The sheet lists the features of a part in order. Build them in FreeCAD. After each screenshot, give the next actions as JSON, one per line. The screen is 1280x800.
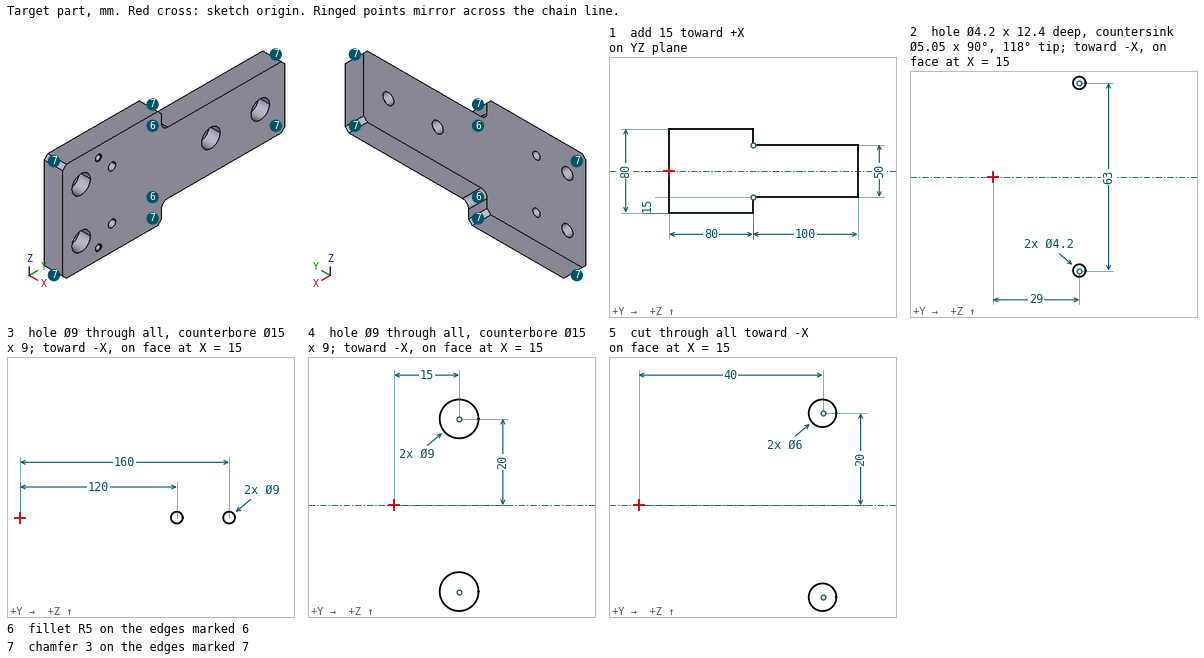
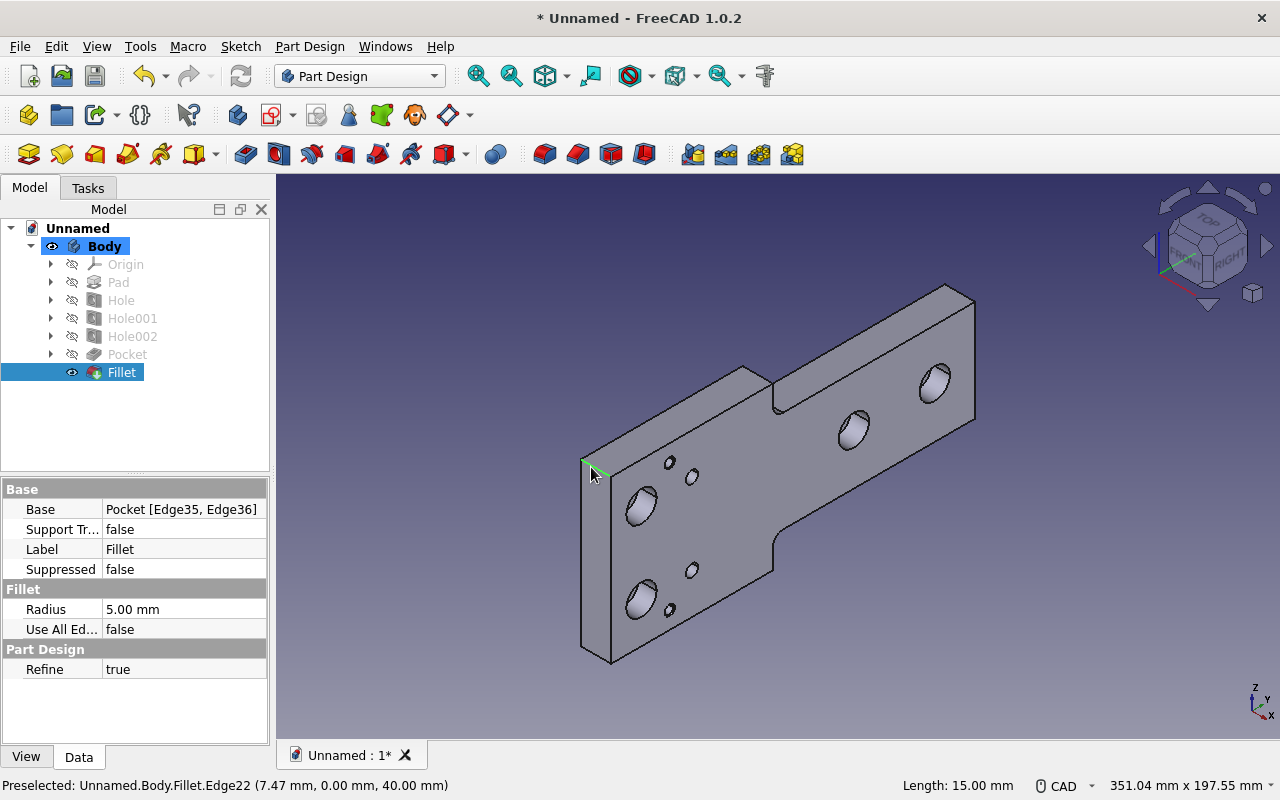
{"action": "key", "text": "2"}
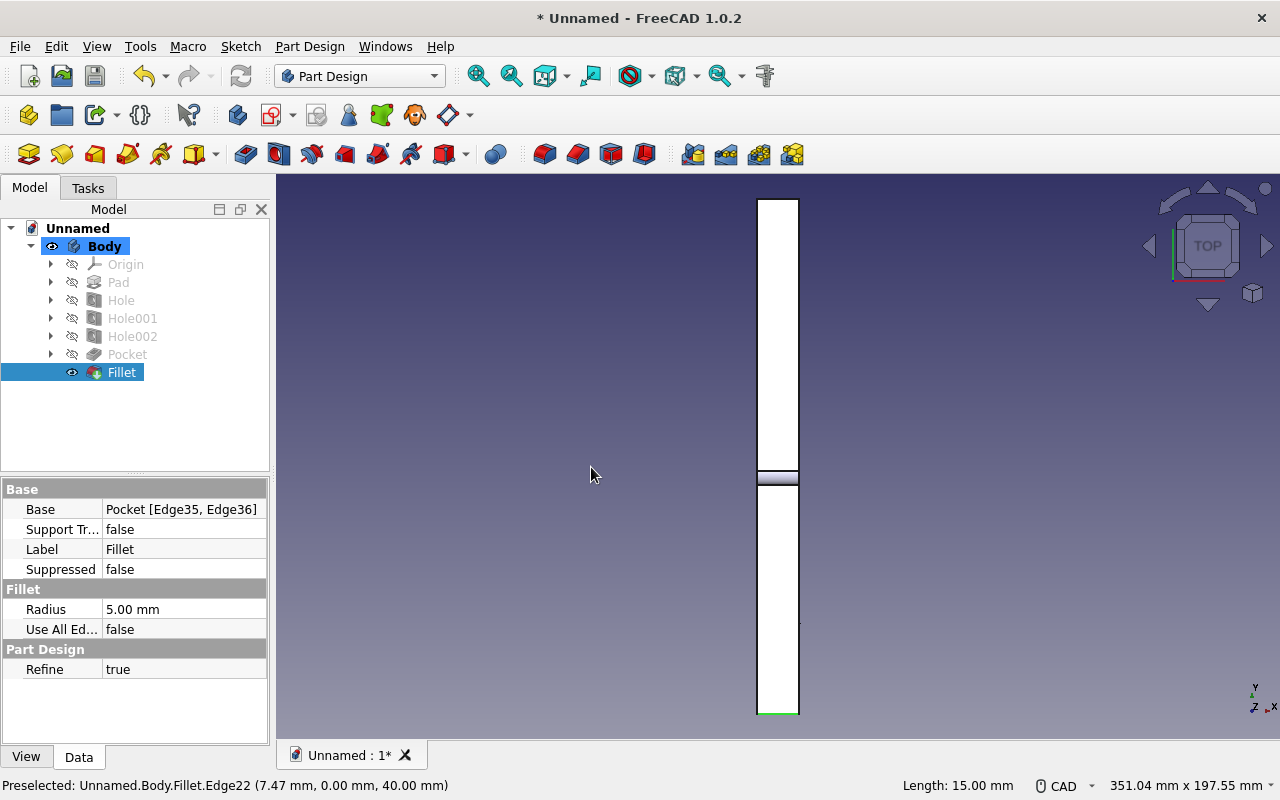
{"action": "left_click", "coordinate": [778, 484], "text": "ctrl"}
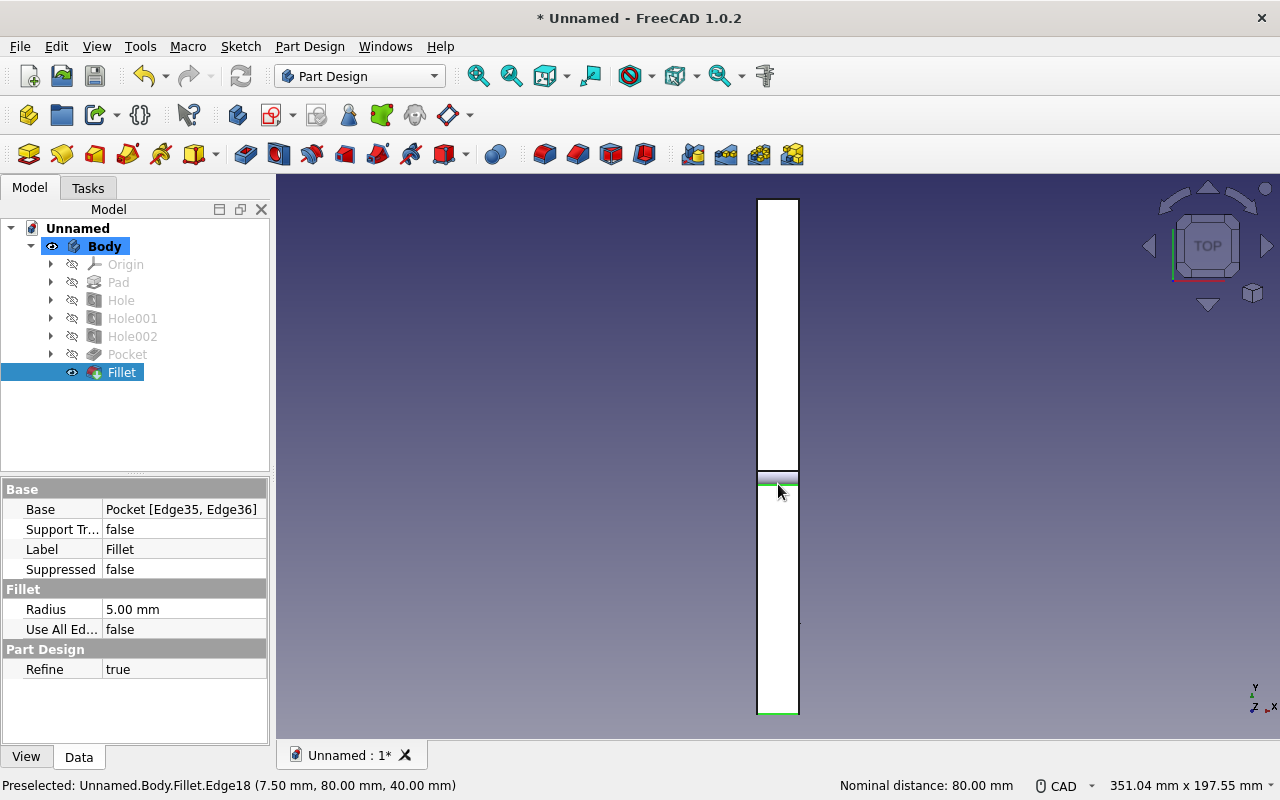
{"action": "key", "text": "0"}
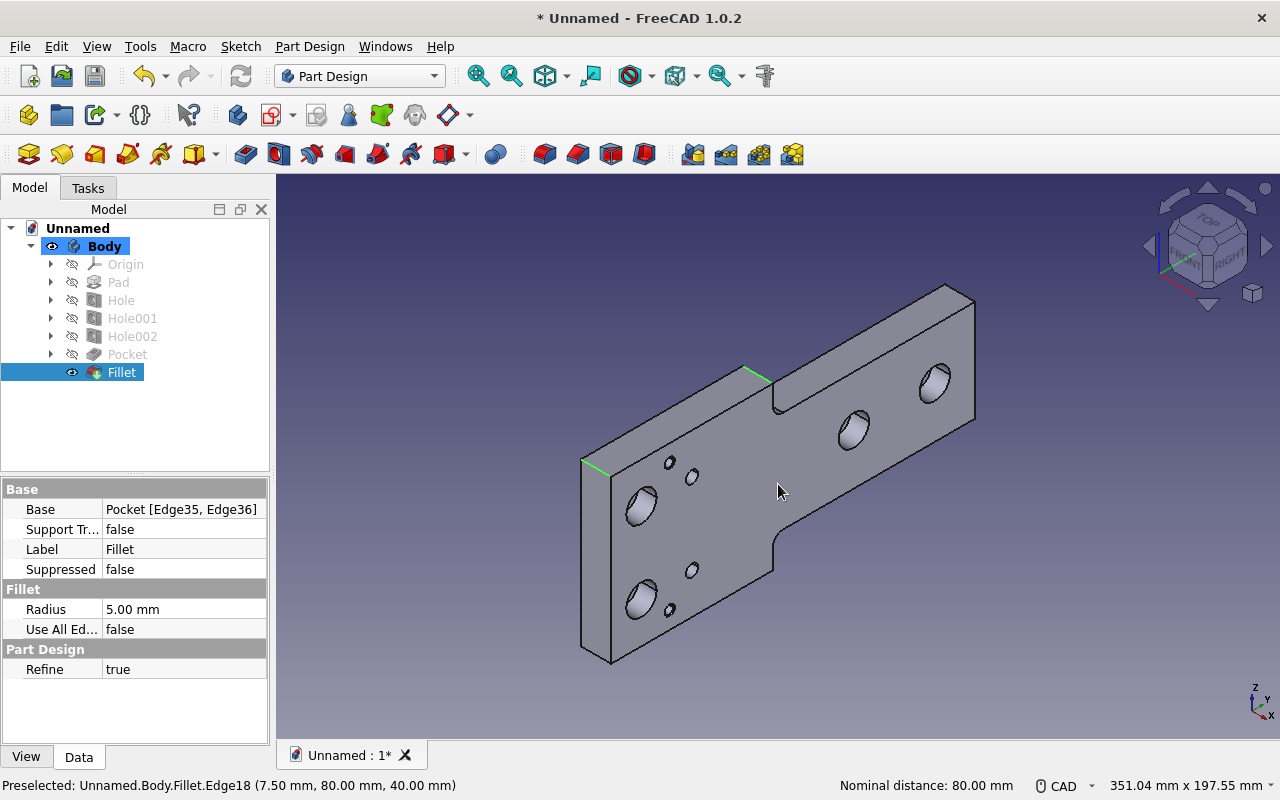
{"action": "key", "text": "1"}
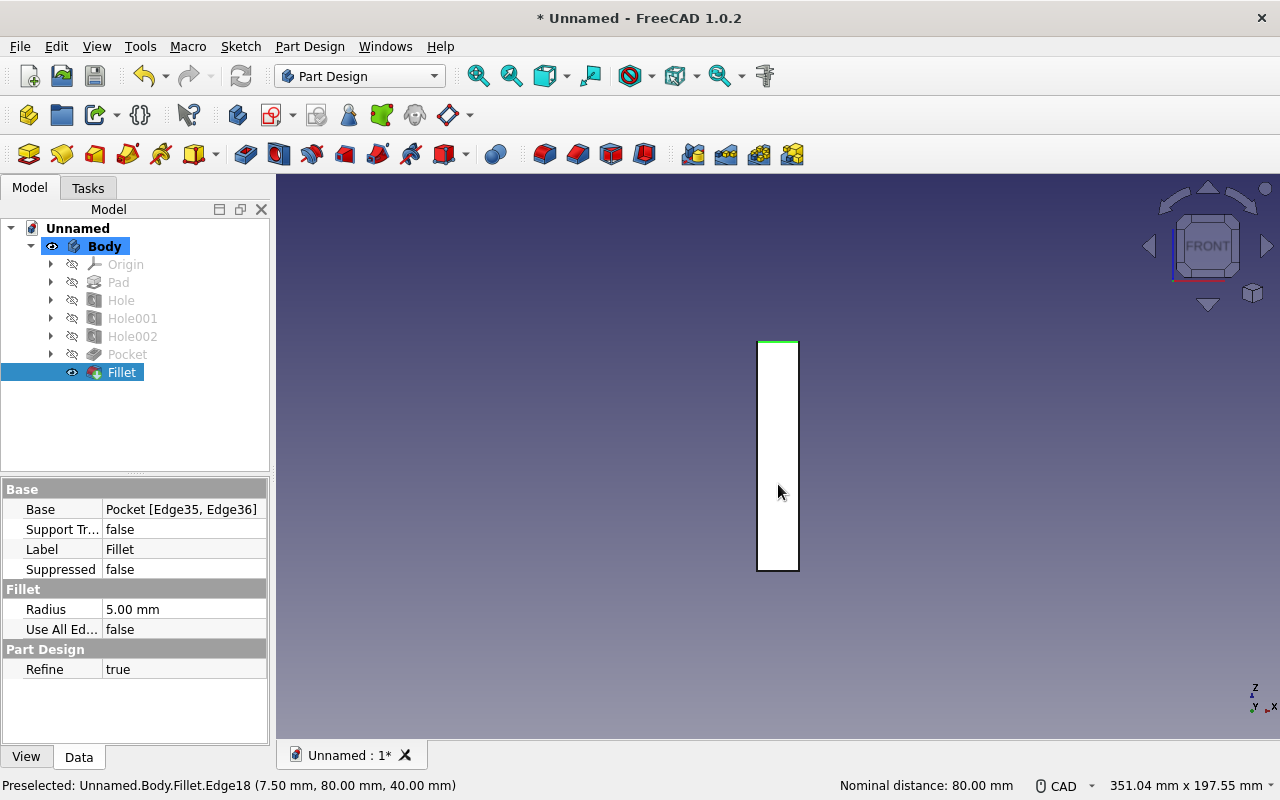
{"action": "left_click", "coordinate": [479, 76]}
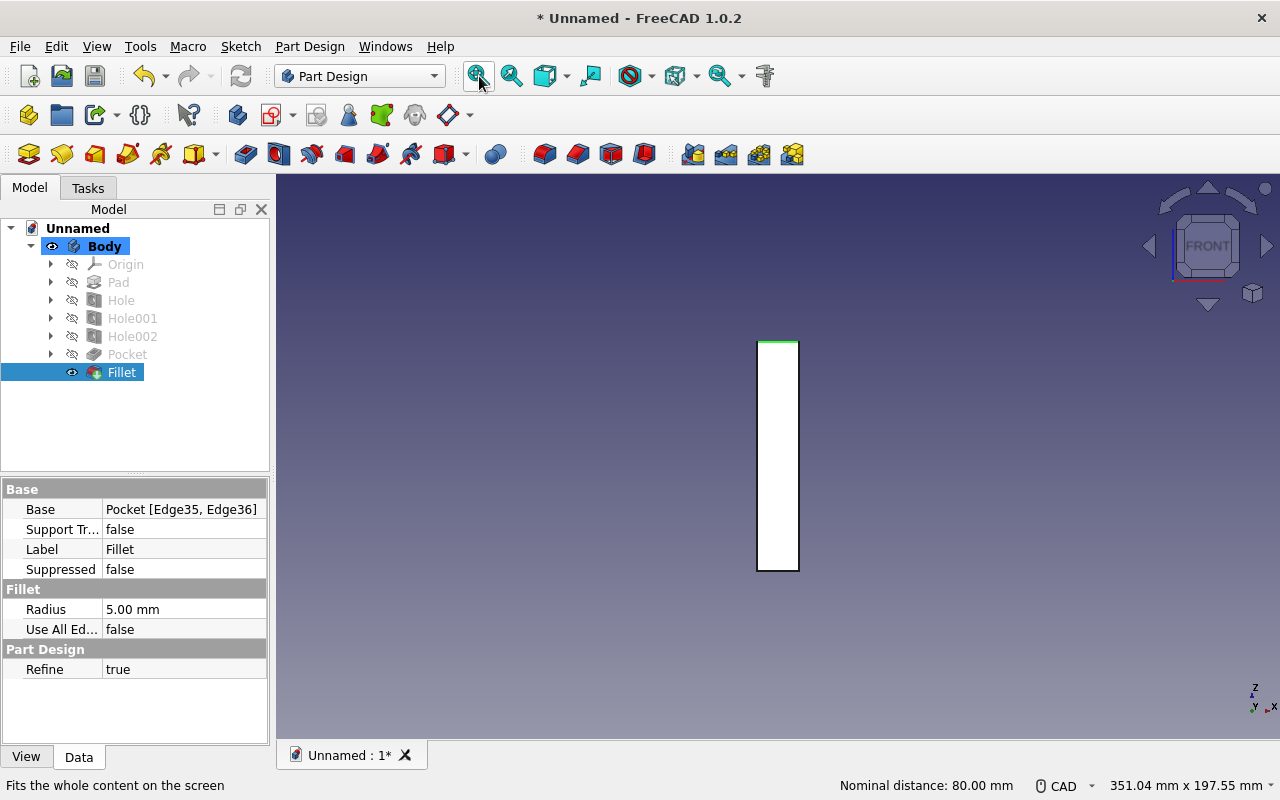
{"action": "left_click", "coordinate": [778, 570], "text": "ctrl"}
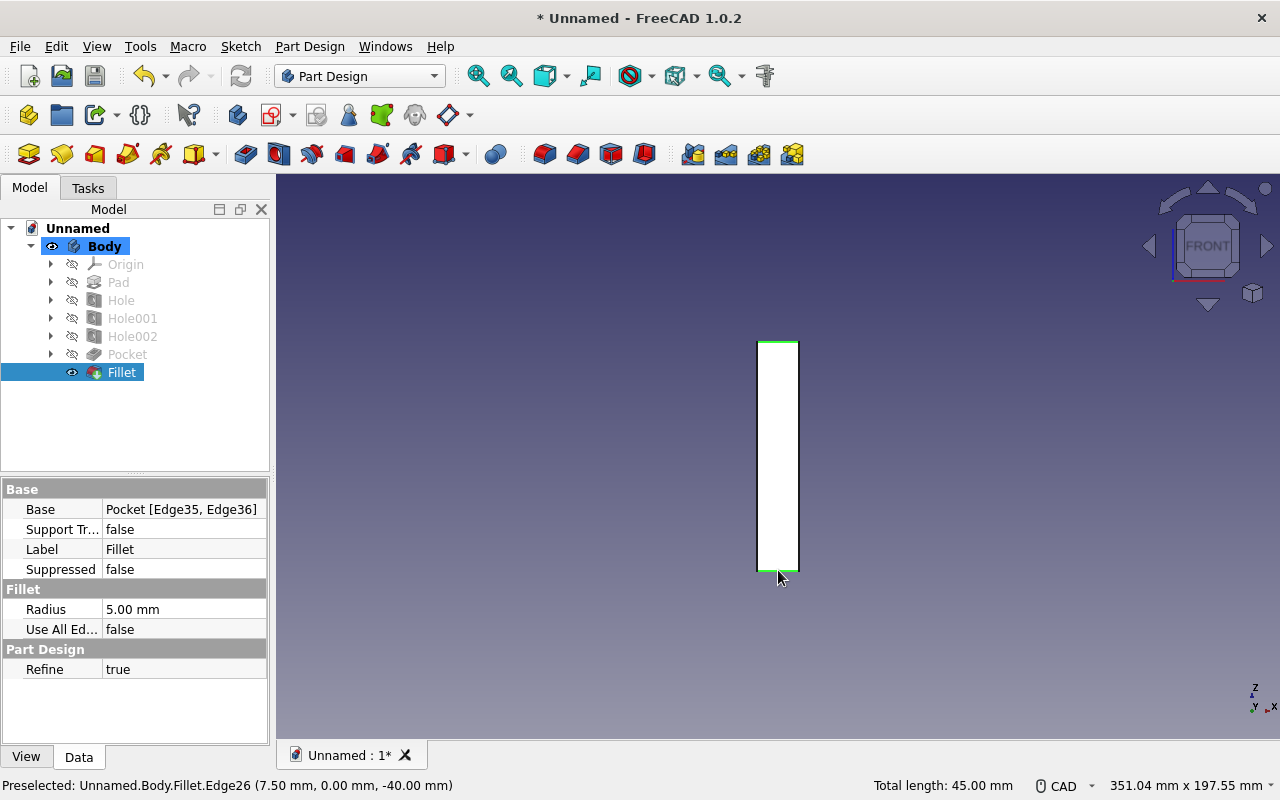
{"action": "key", "text": "3"}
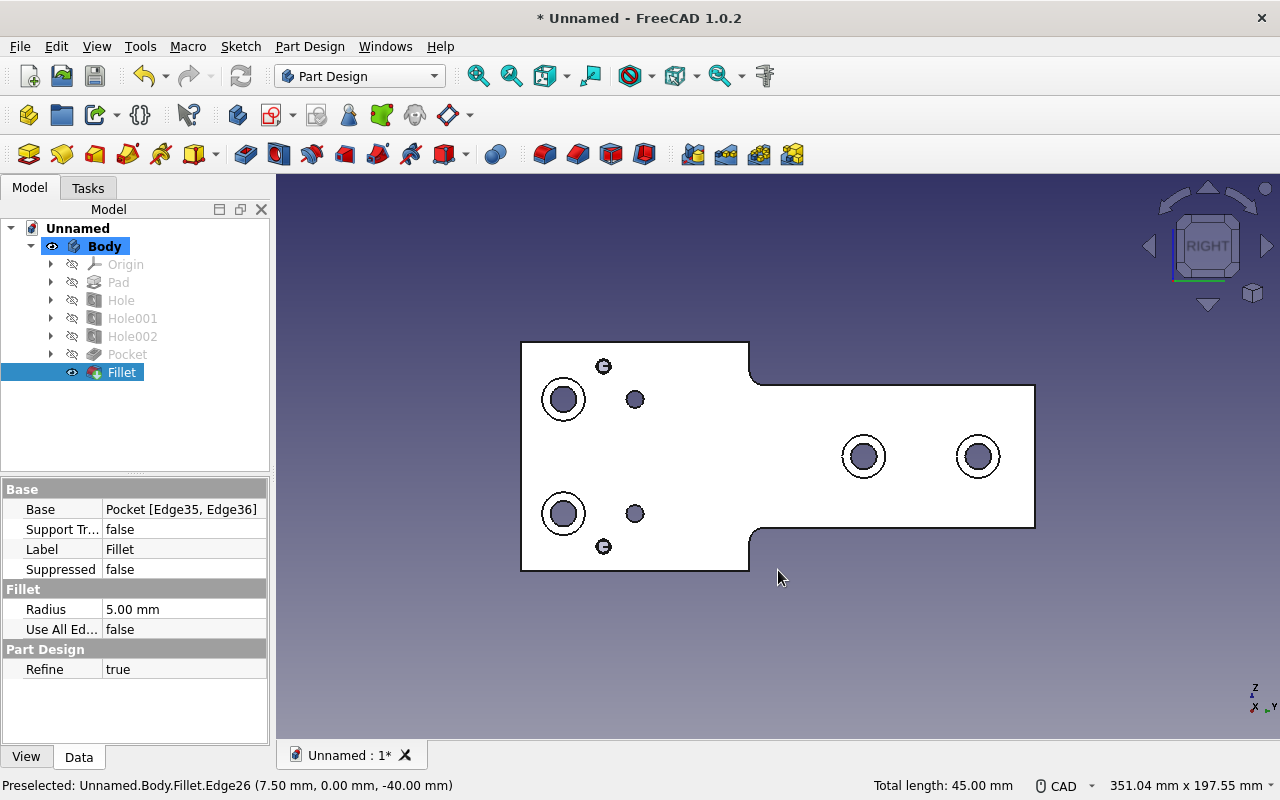
{"action": "key", "text": "5"}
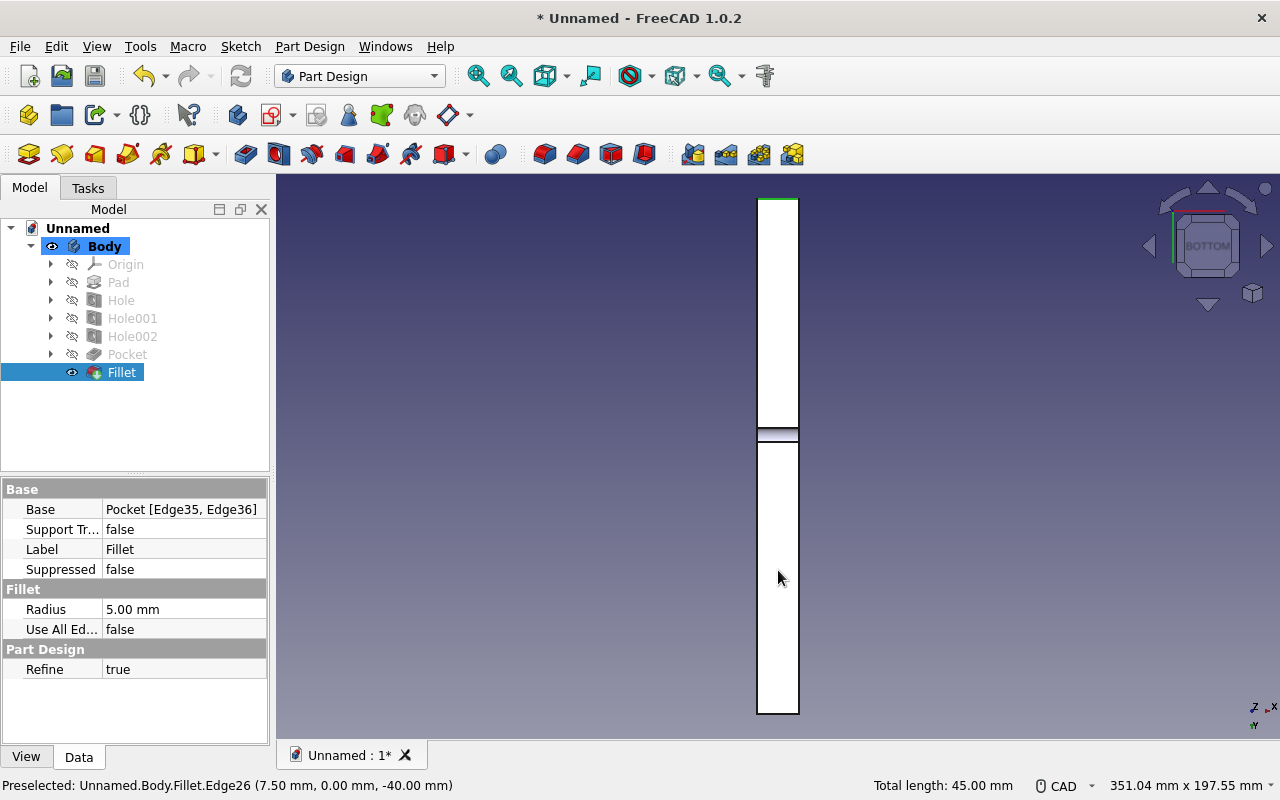
{"action": "left_click", "coordinate": [778, 427], "text": "ctrl"}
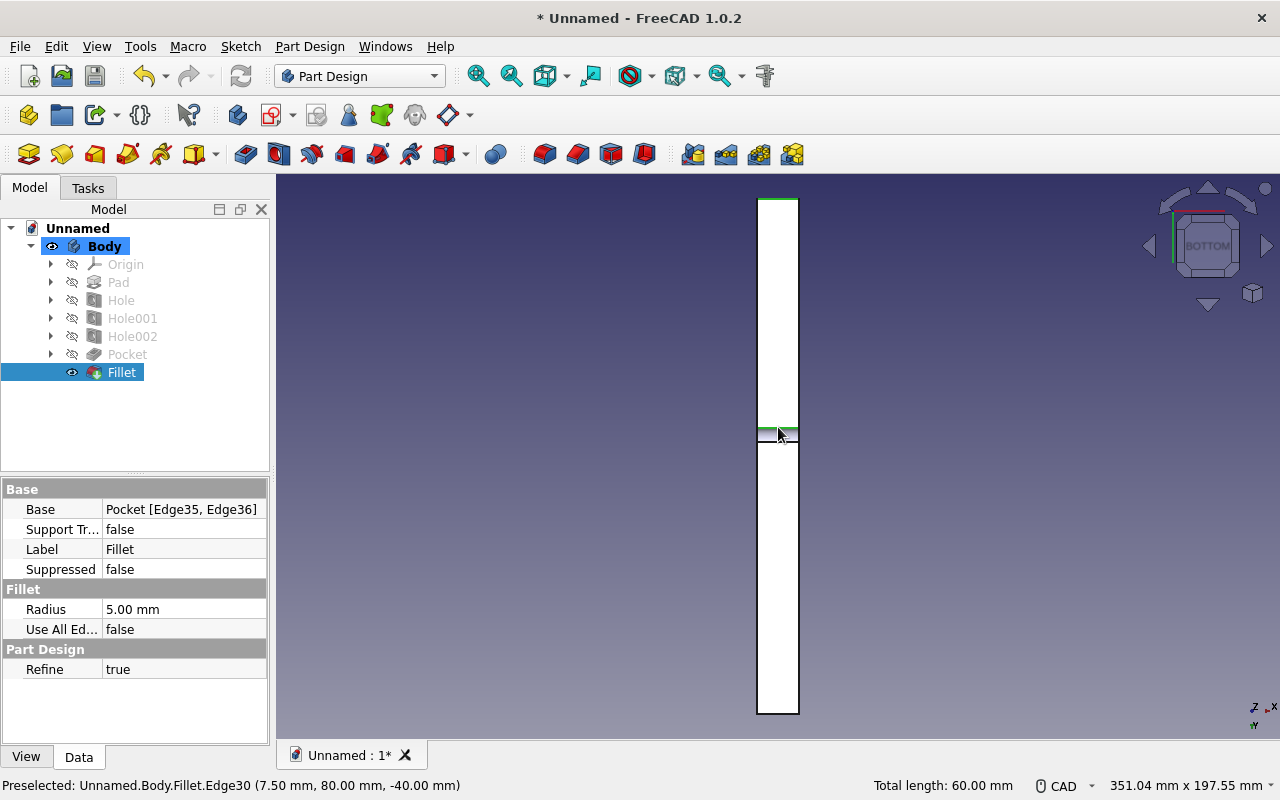
{"action": "key", "text": "4"}